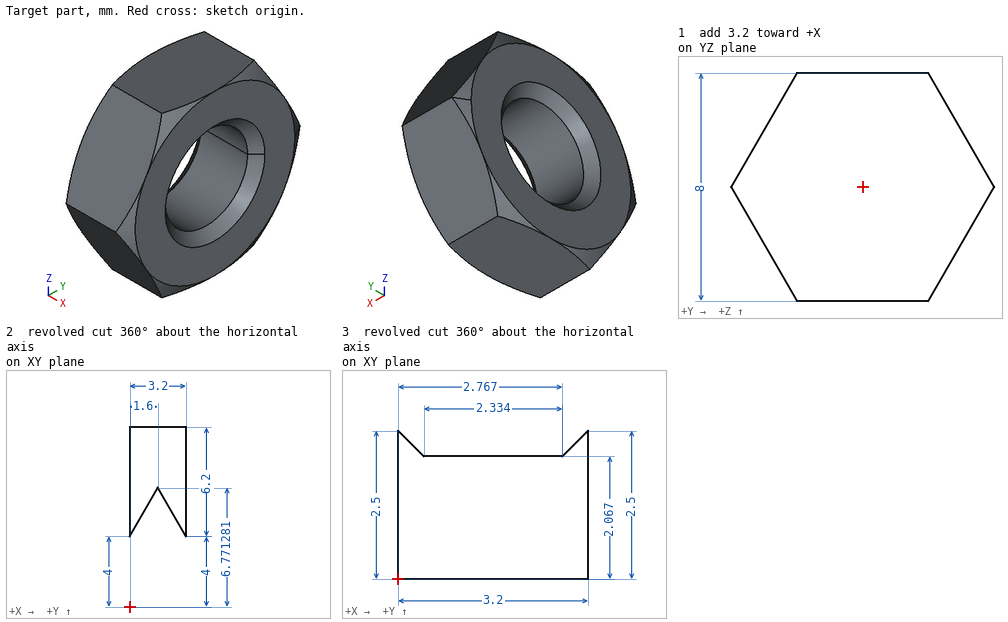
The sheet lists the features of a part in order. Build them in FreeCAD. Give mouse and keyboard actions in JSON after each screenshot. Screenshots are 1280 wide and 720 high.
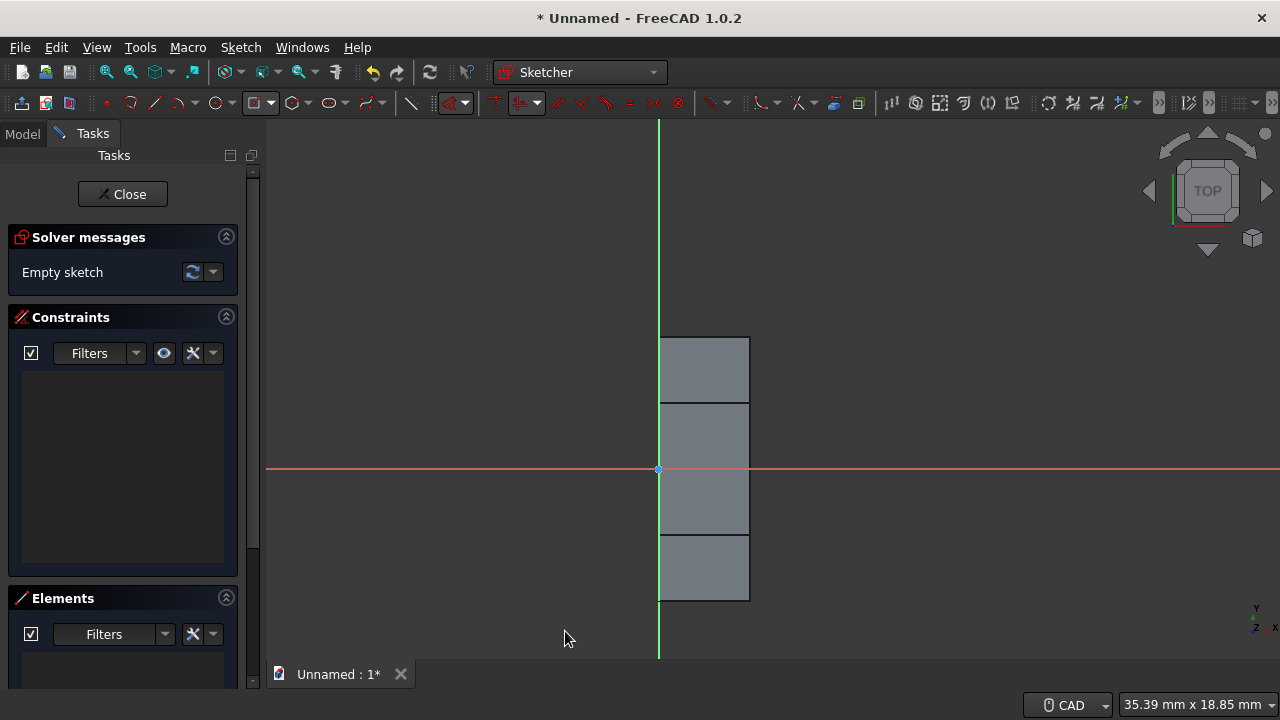
{"action": "key", "text": "g m"}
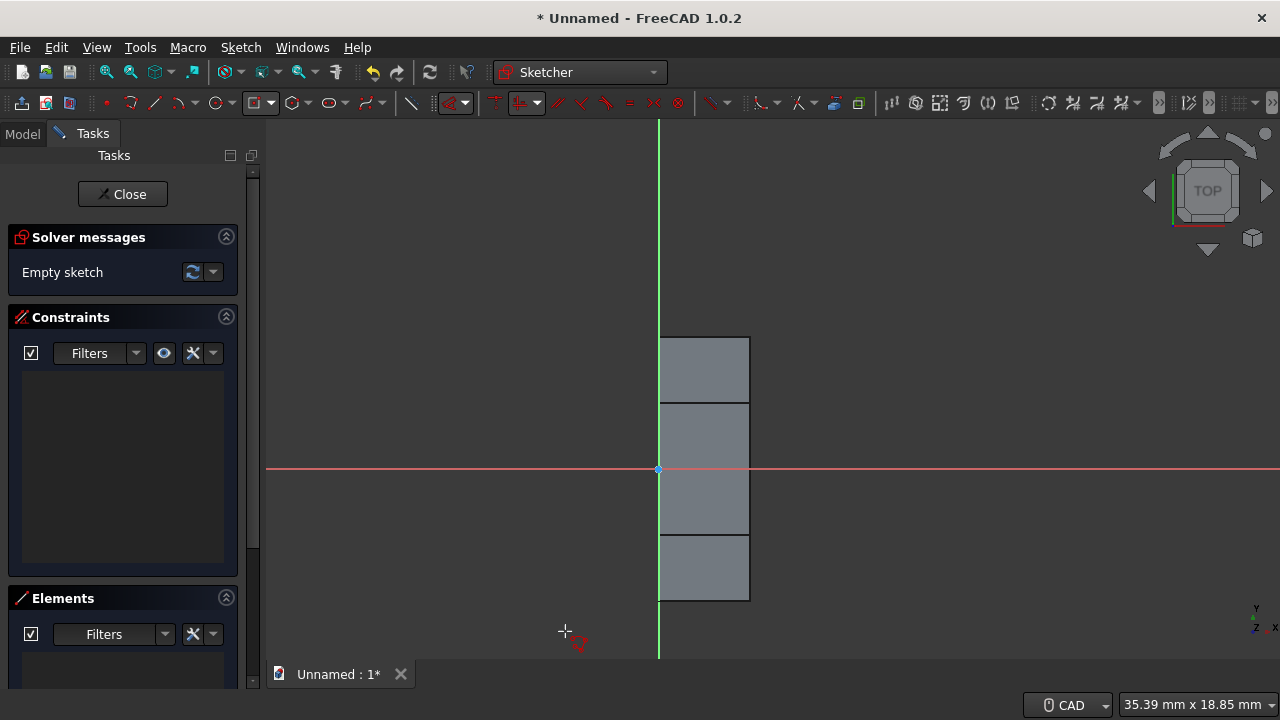
{"action": "left_click", "coordinate": [659, 354]}
{"action": "left_click", "coordinate": [705, 275]}
{"action": "left_click", "coordinate": [750, 354]}
{"action": "left_click", "coordinate": [750, 177]}
{"action": "left_click", "coordinate": [668, 177]}
{"action": "left_click", "coordinate": [659, 355]}
{"action": "key", "text": "Escape"}
{"action": "key", "text": "Escape"}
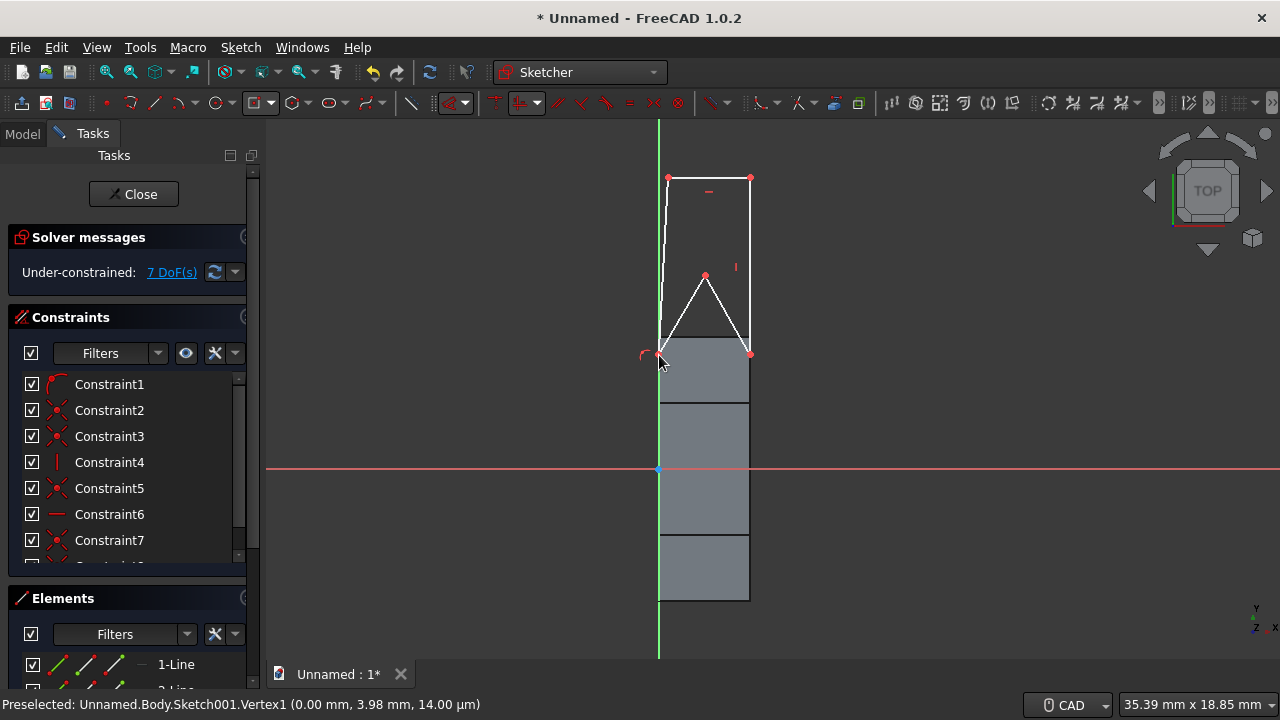
{"action": "left_click", "coordinate": [661, 302]}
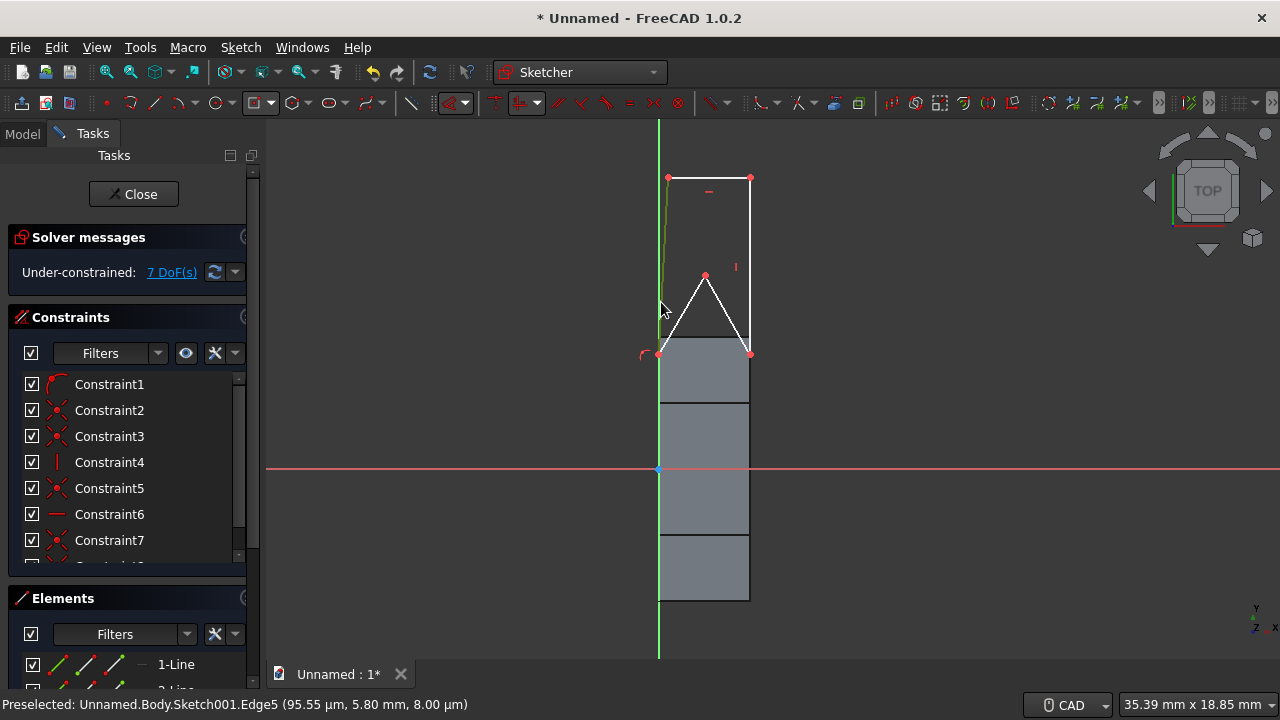
{"action": "key", "text": "v"}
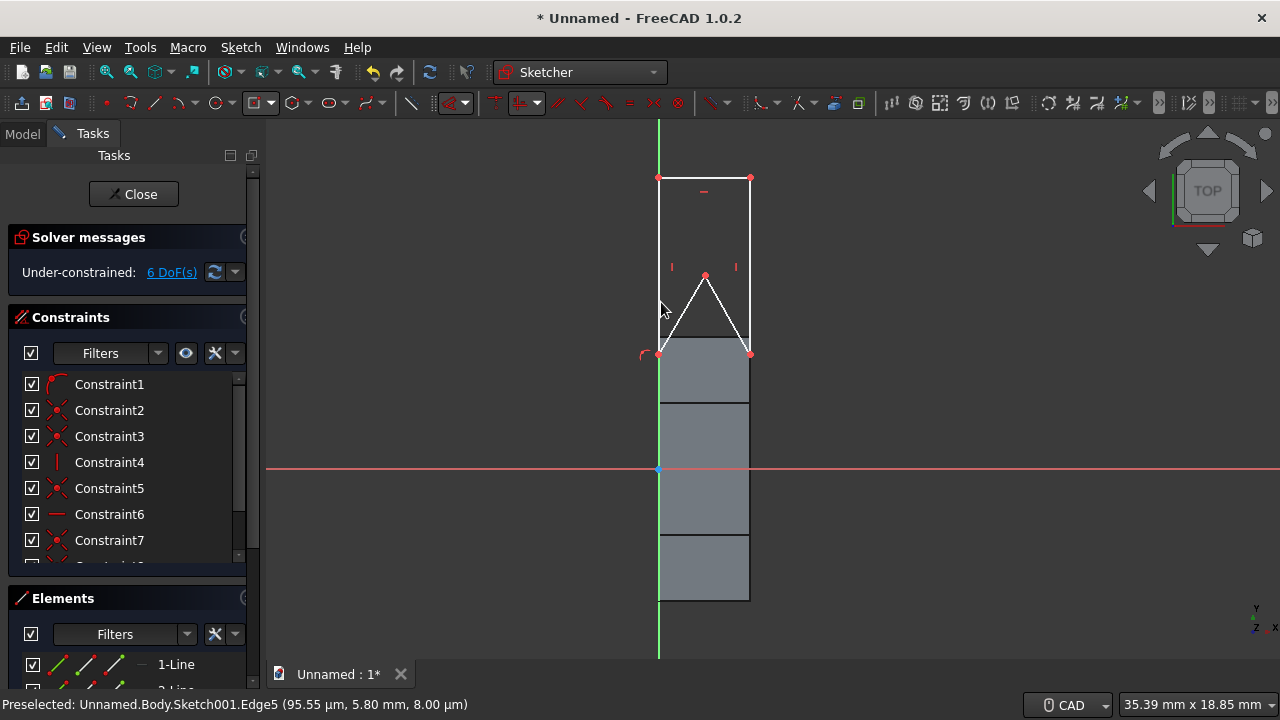
{"action": "left_click", "coordinate": [450, 104]}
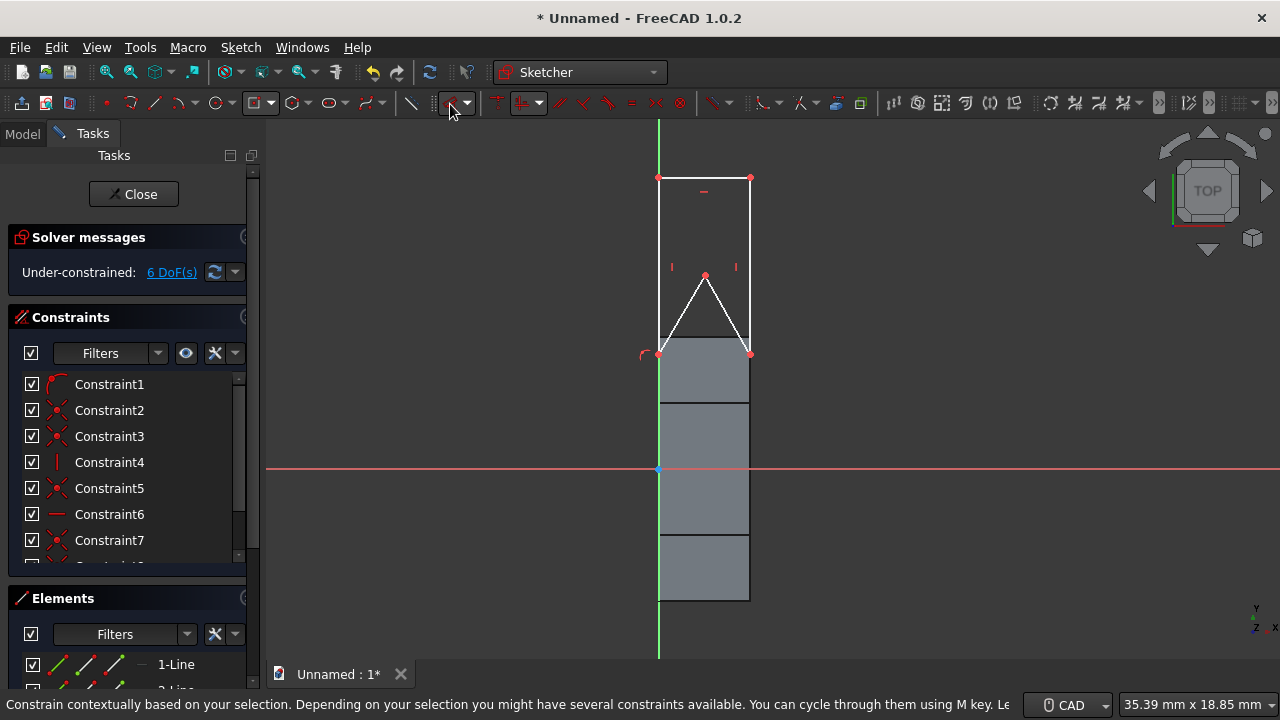
{"action": "left_click", "coordinate": [659, 355]}
{"action": "left_click", "coordinate": [625, 412]}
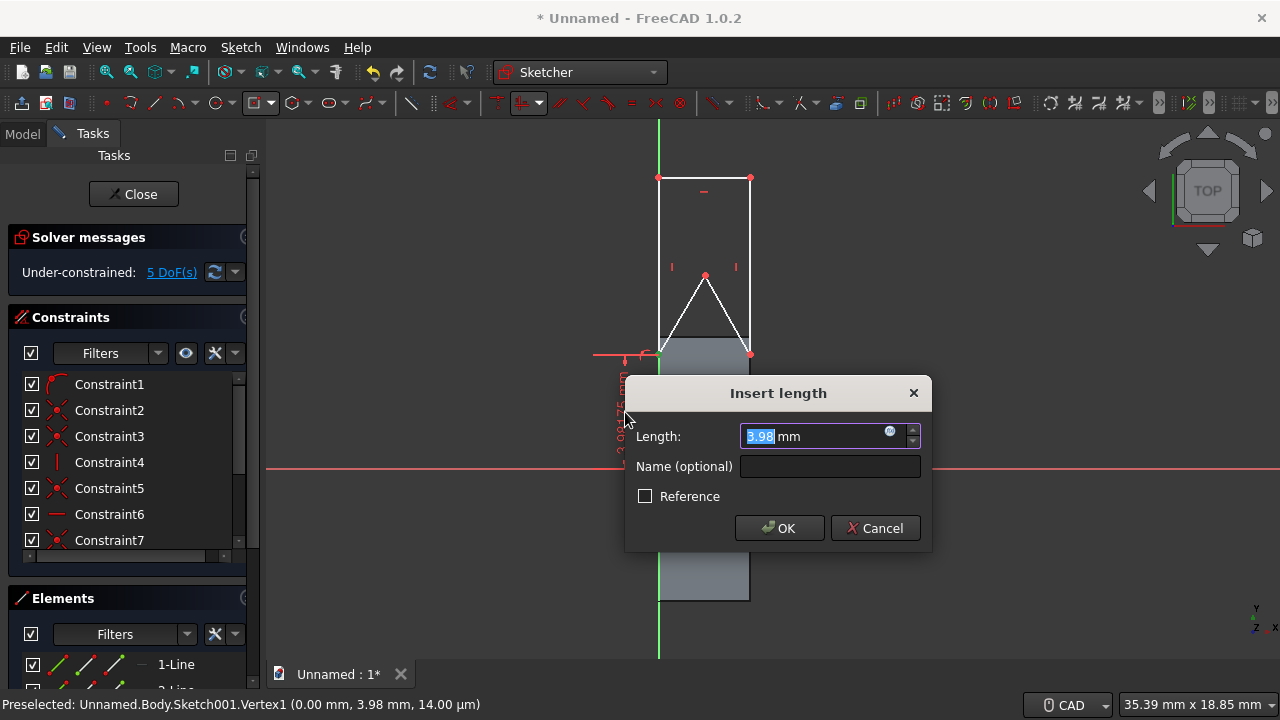
{"action": "type", "text": "4"}
{"action": "key", "text": "Return"}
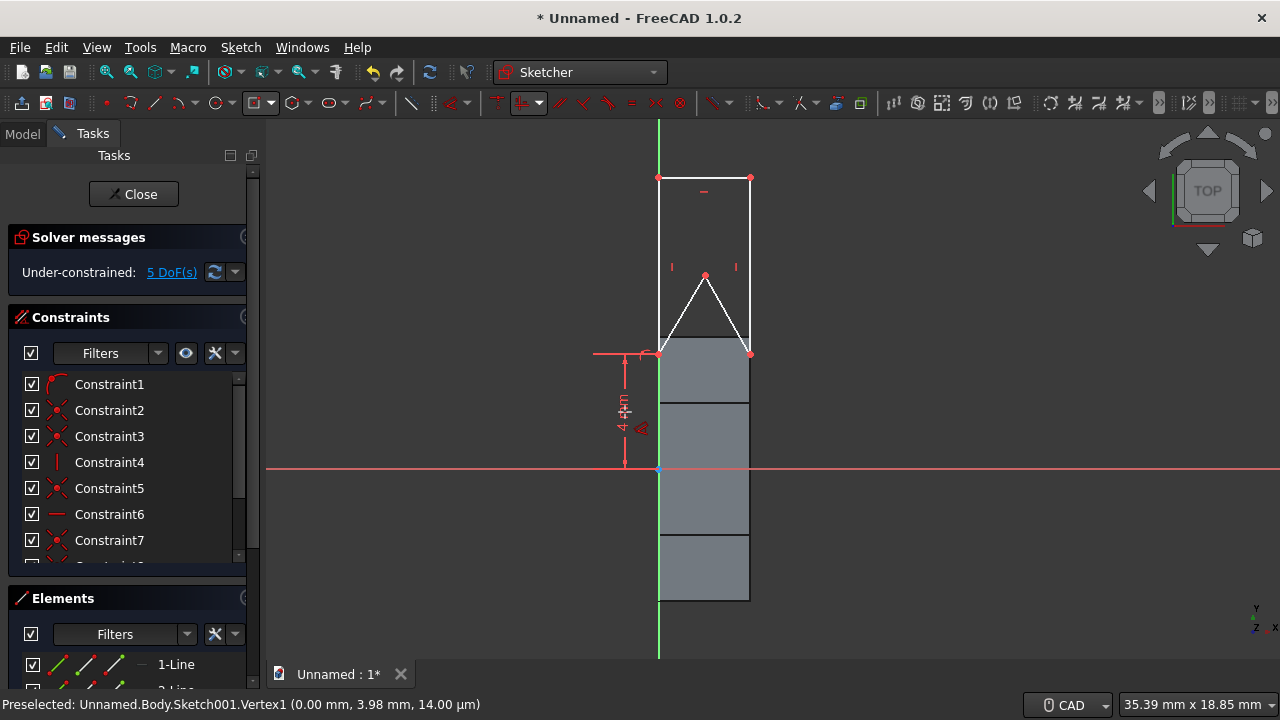
{"action": "left_click", "coordinate": [750, 355]}
{"action": "left_click", "coordinate": [625, 386]}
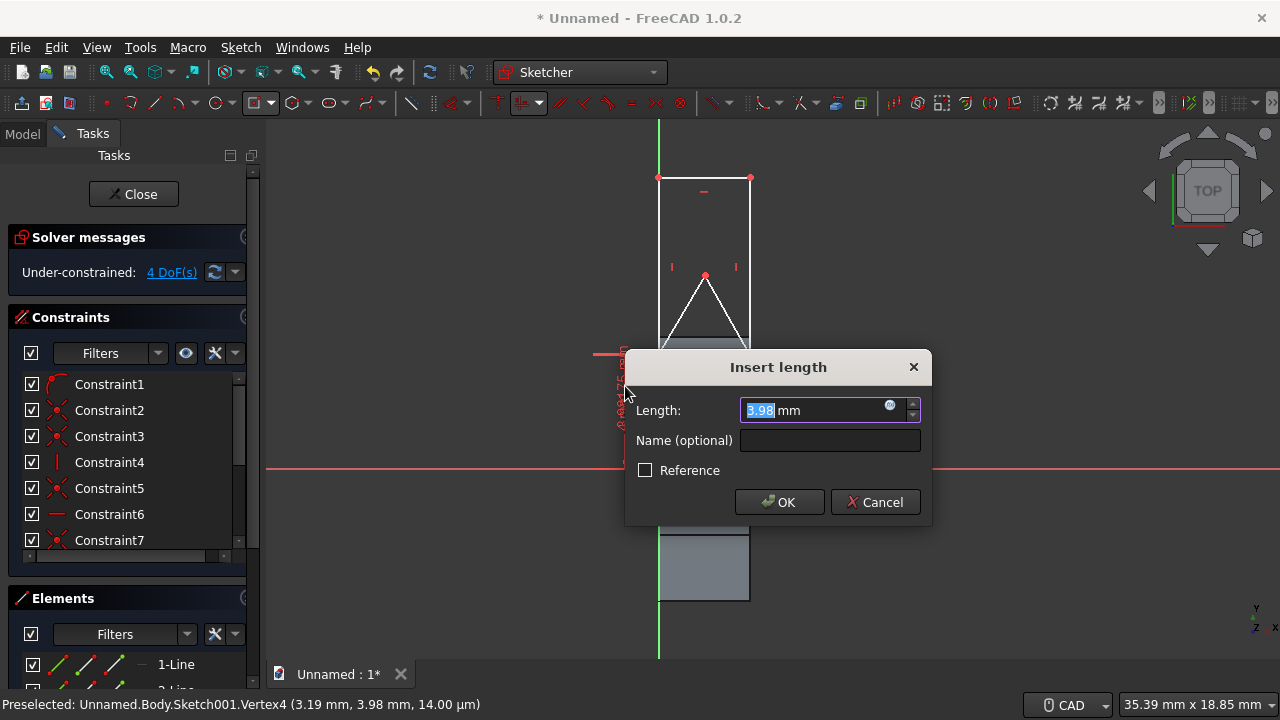
{"action": "type", "text": "4"}
{"action": "key", "text": "Return"}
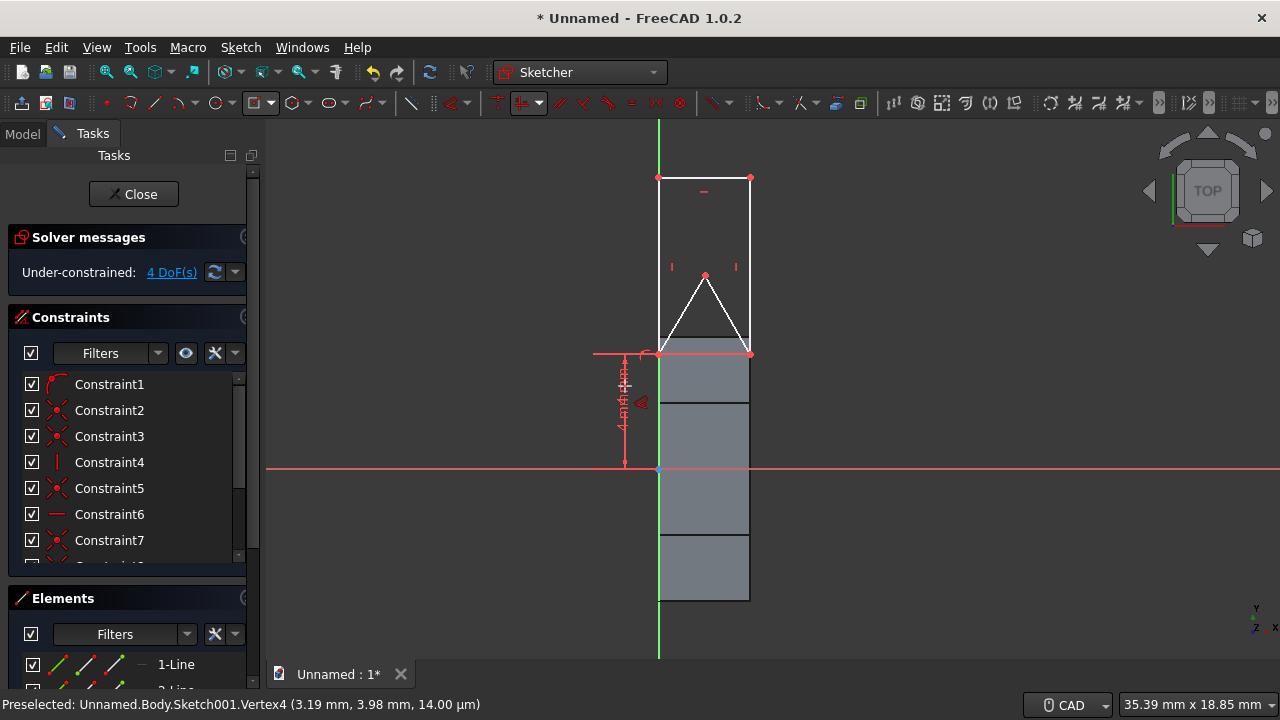
{"action": "left_click", "coordinate": [750, 302]}
{"action": "left_click", "coordinate": [784, 266]}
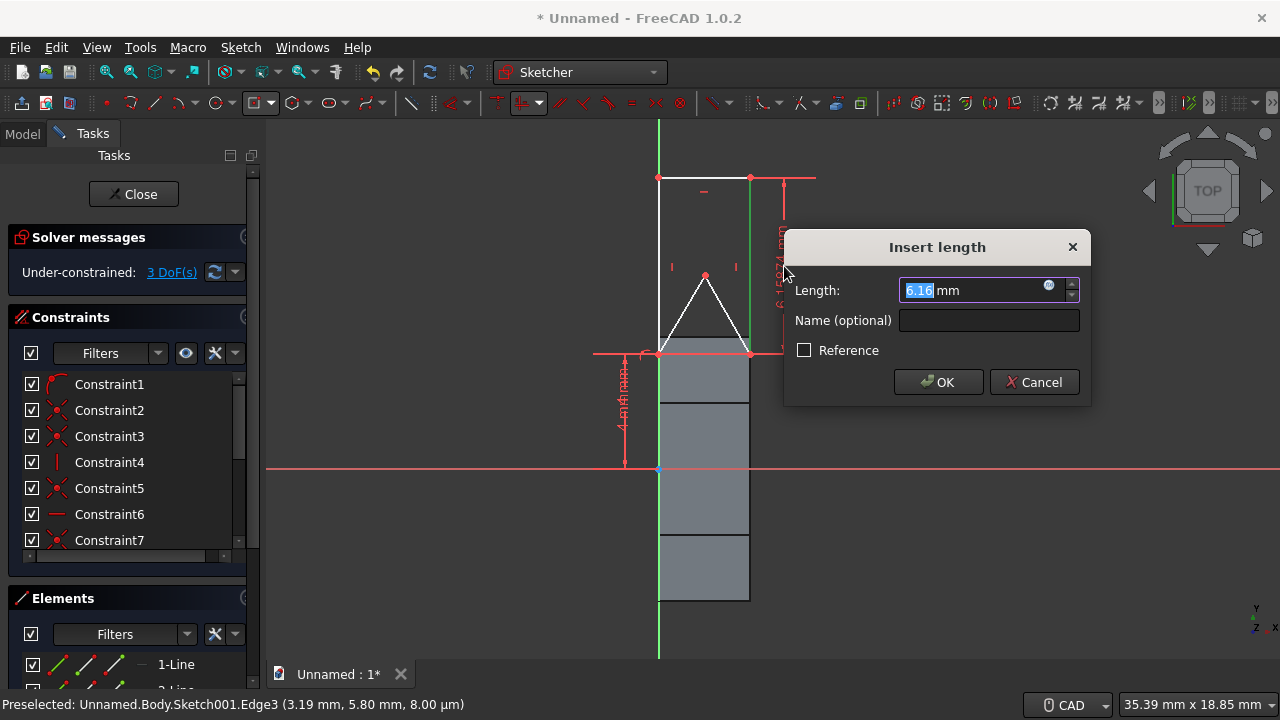
{"action": "type", "text": "6.2"}
{"action": "key", "text": "Return"}